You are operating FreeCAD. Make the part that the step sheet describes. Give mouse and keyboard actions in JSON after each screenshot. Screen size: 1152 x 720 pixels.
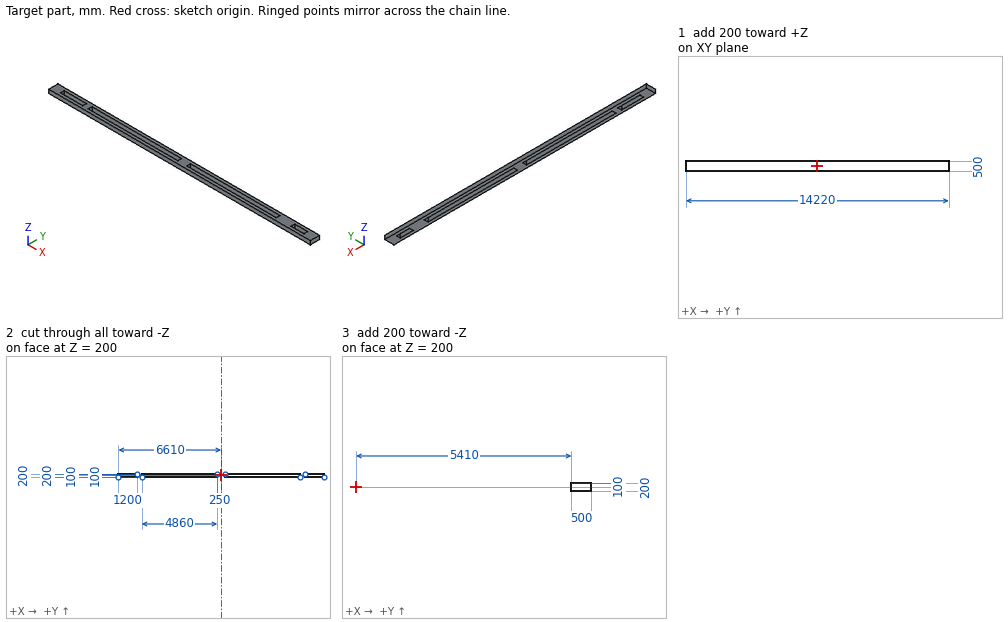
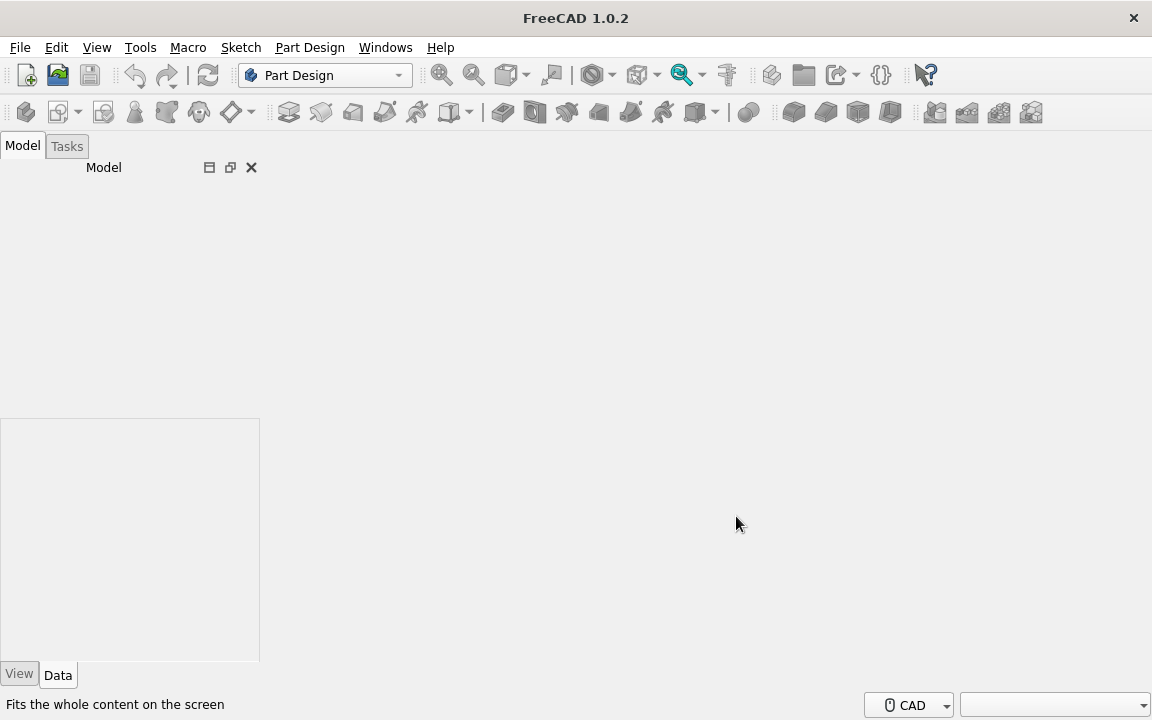
{"action": "left_click", "coordinate": [26, 76]}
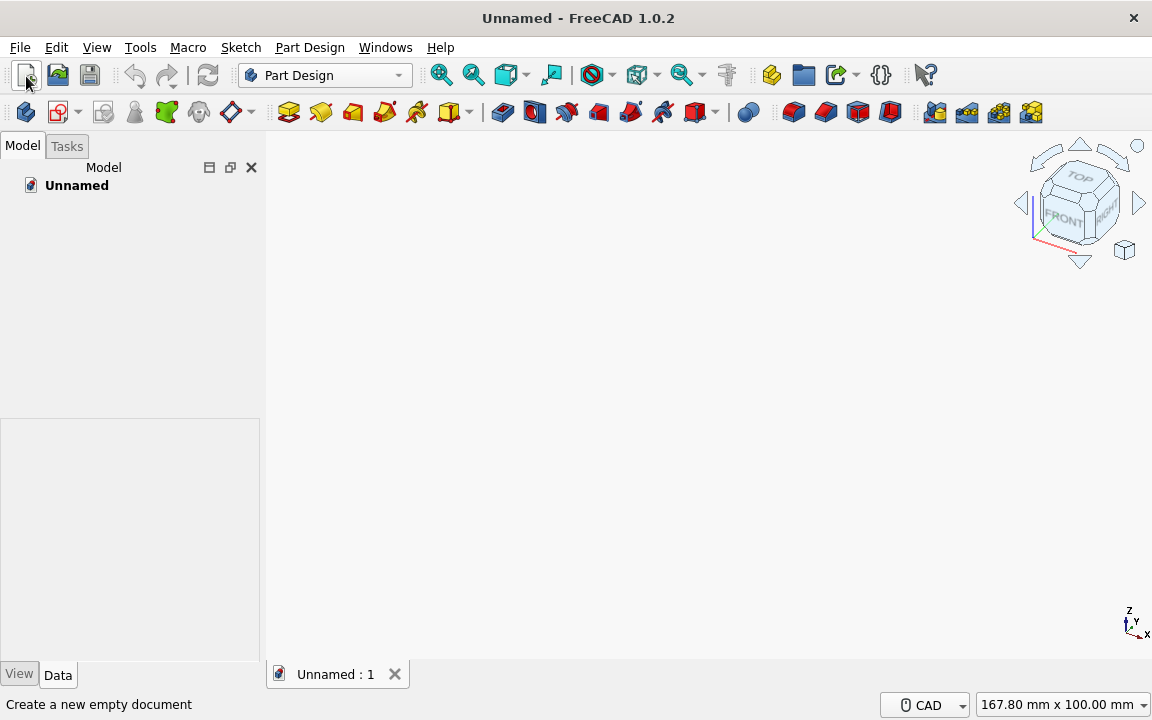
{"action": "left_click", "coordinate": [58, 112]}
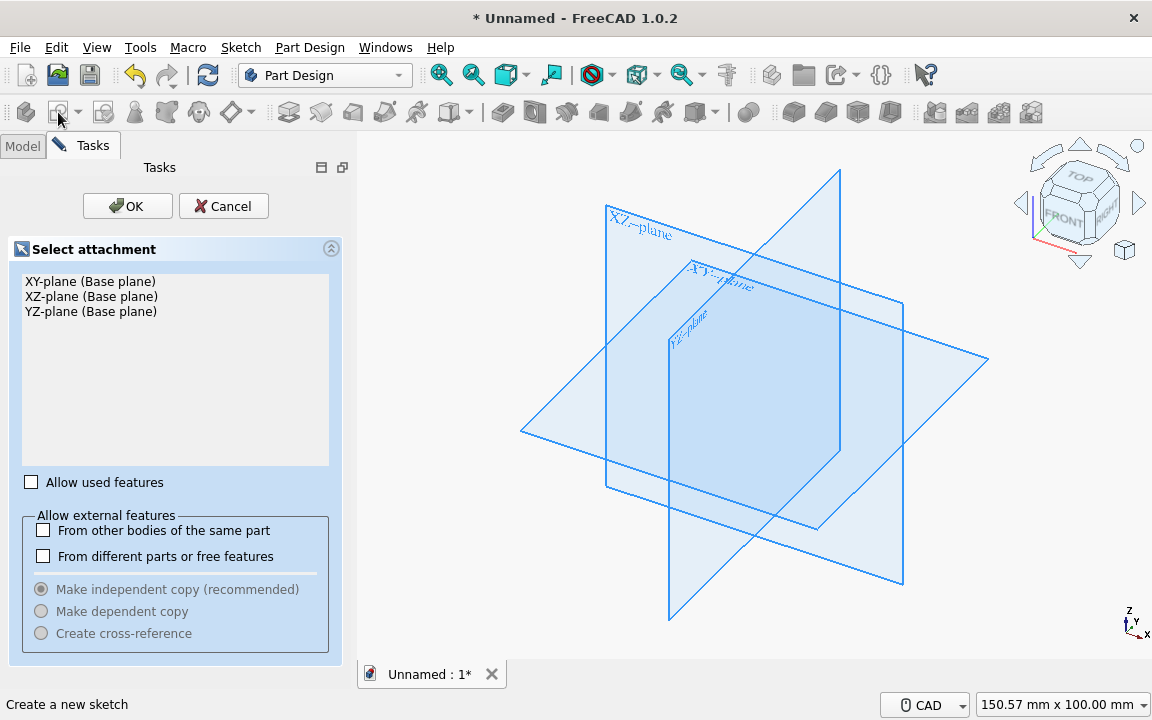
{"action": "left_click", "coordinate": [82, 282]}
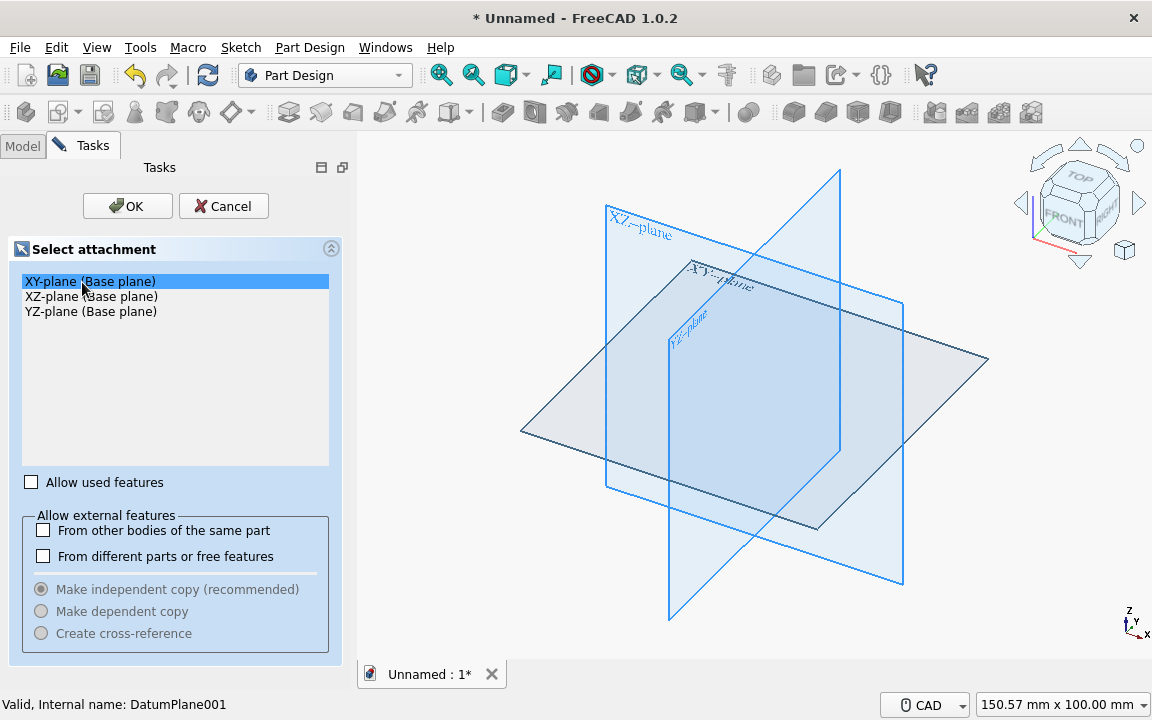
{"action": "left_click", "coordinate": [128, 206]}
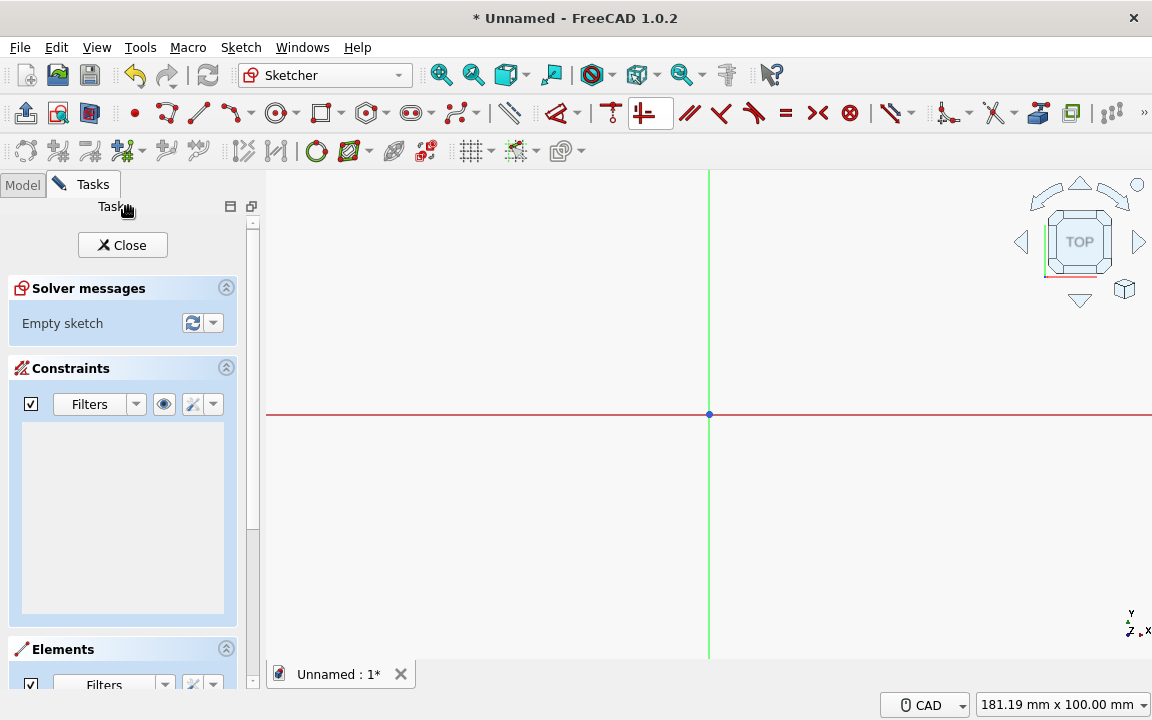
{"action": "scroll", "coordinate": [640, 414], "scroll_direction": "down", "scroll_amount": 15}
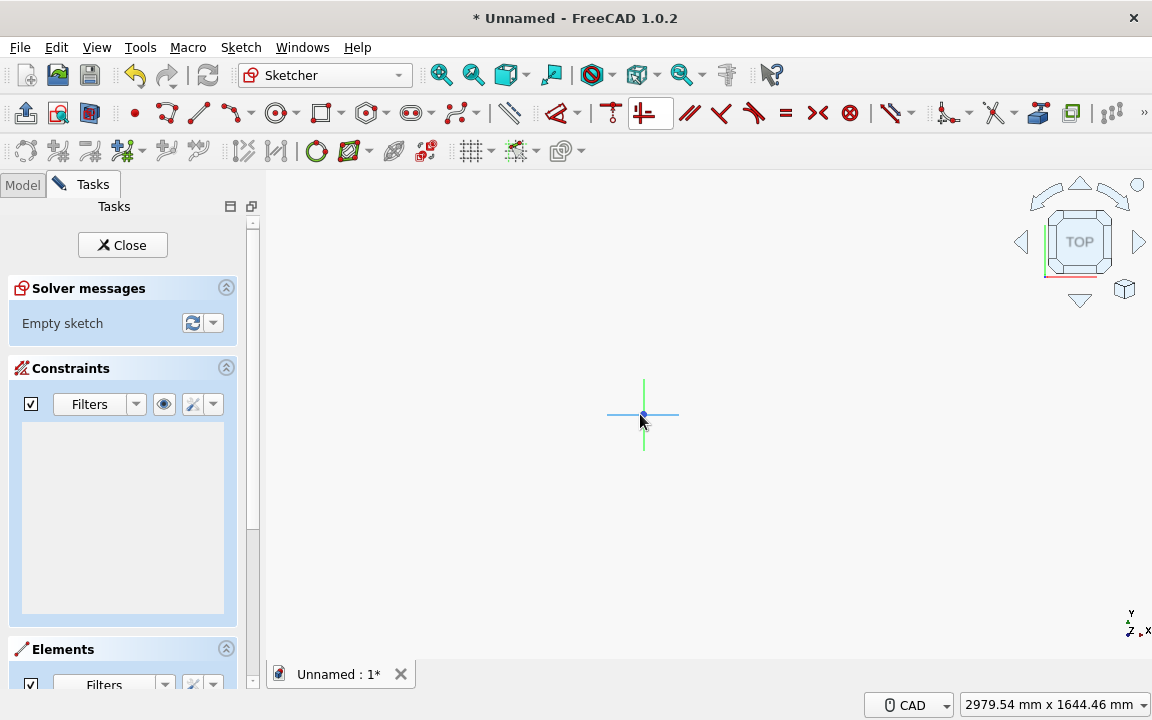
{"action": "scroll", "coordinate": [640, 414], "scroll_direction": "down", "scroll_amount": 10}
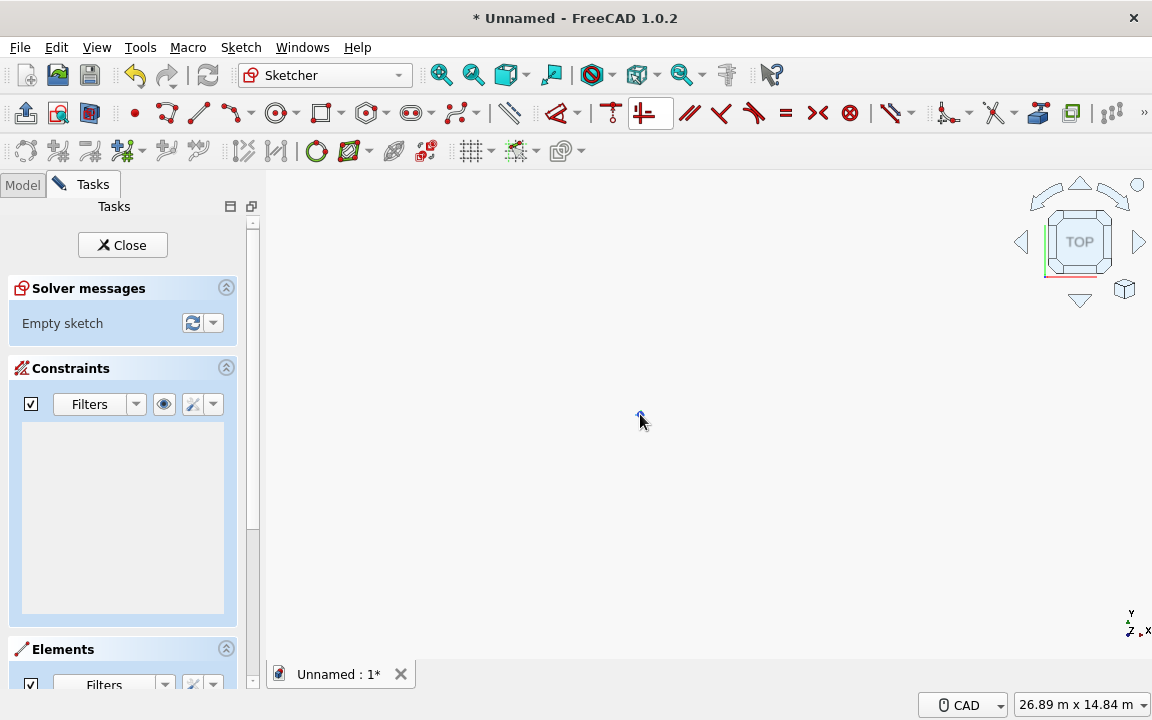
{"action": "left_click", "coordinate": [344, 114]}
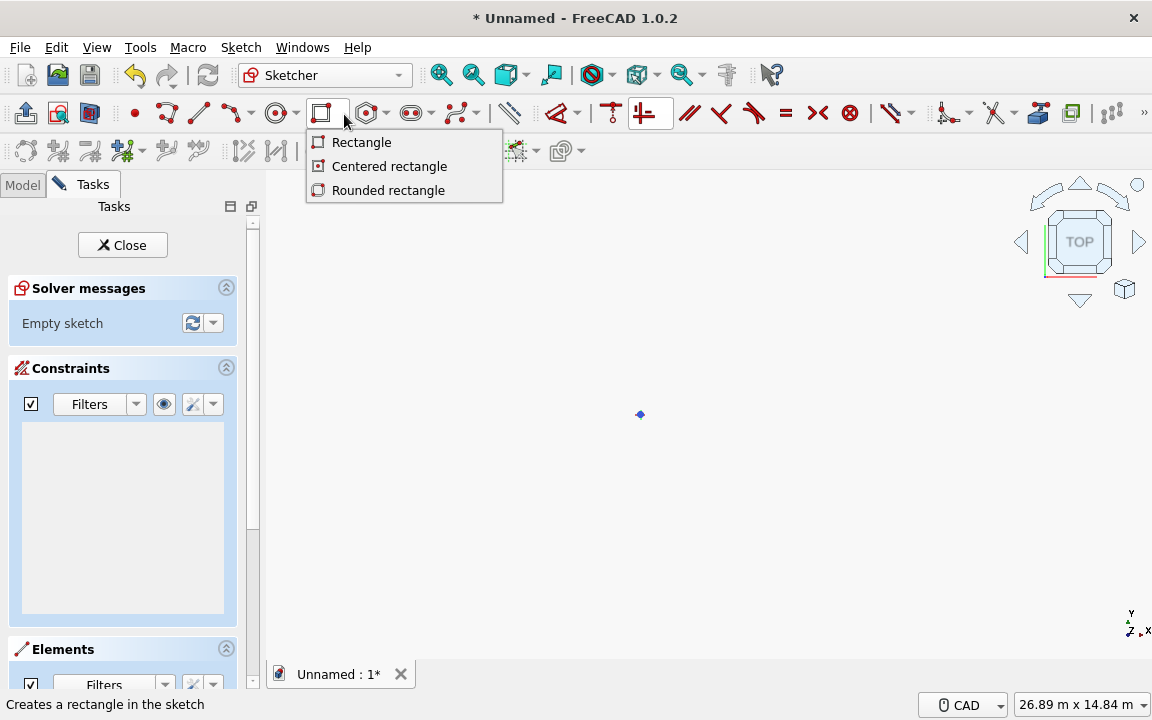
{"action": "left_click", "coordinate": [404, 166]}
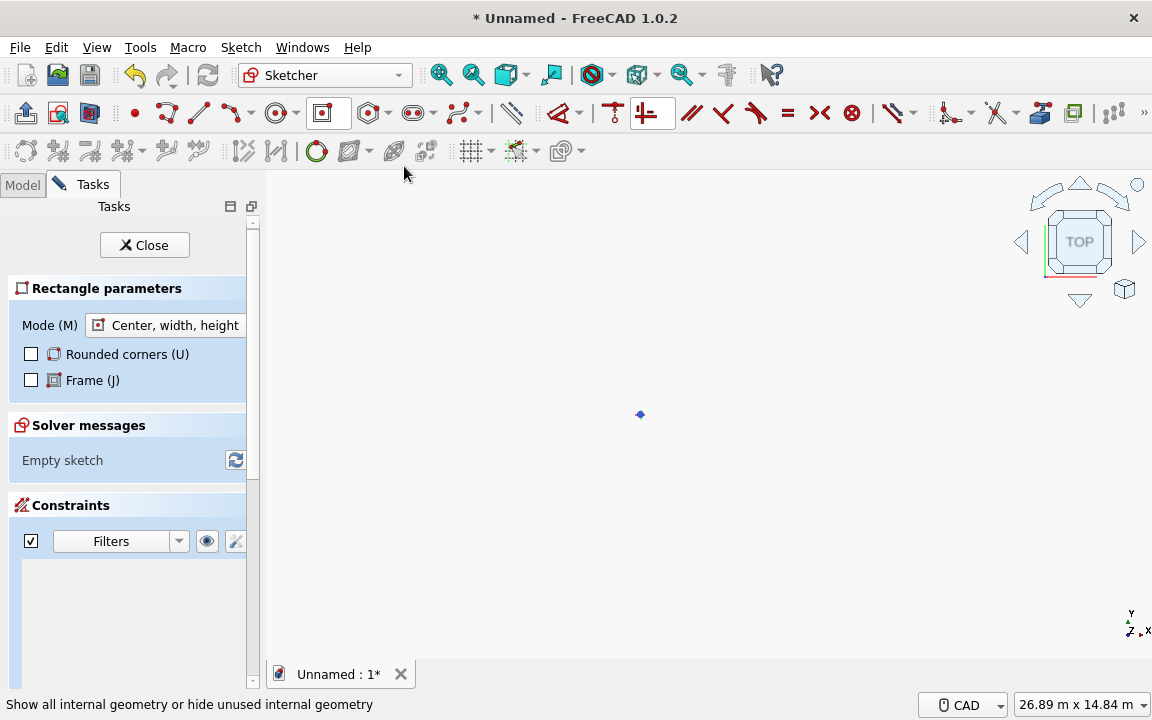
{"action": "scroll", "coordinate": [641, 414], "scroll_direction": "up", "scroll_amount": 4}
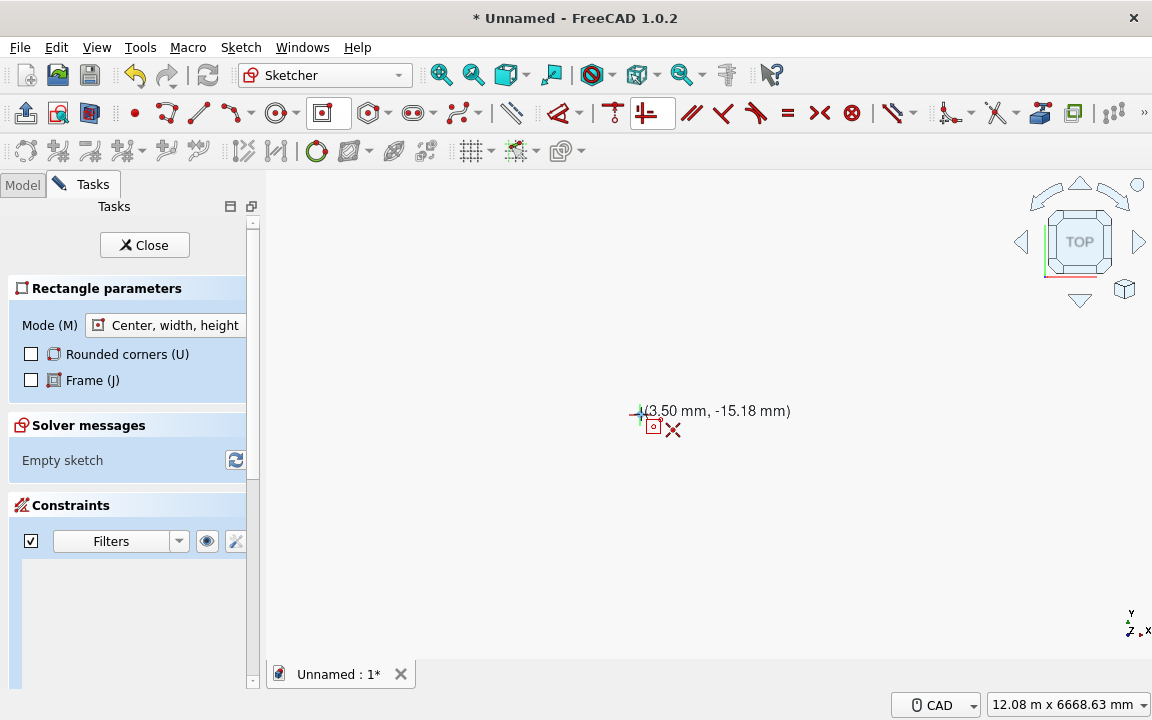
{"action": "left_click", "coordinate": [640, 414]}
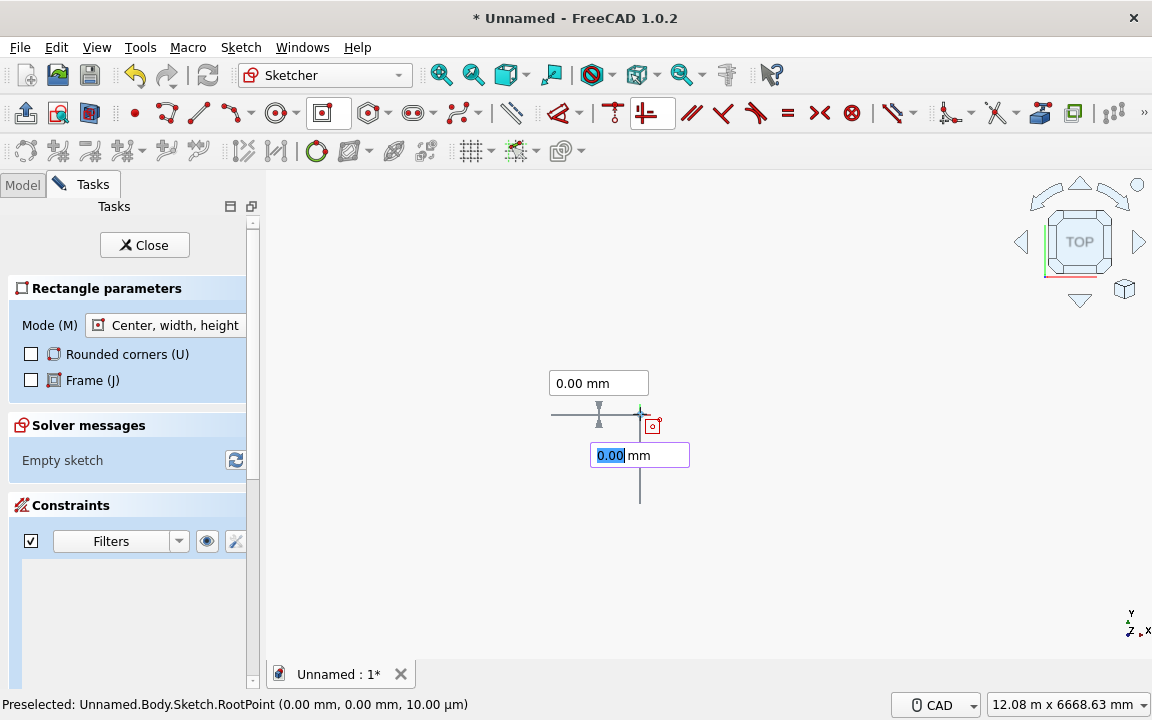
{"action": "scroll", "coordinate": [641, 414], "scroll_direction": "down", "scroll_amount": 4}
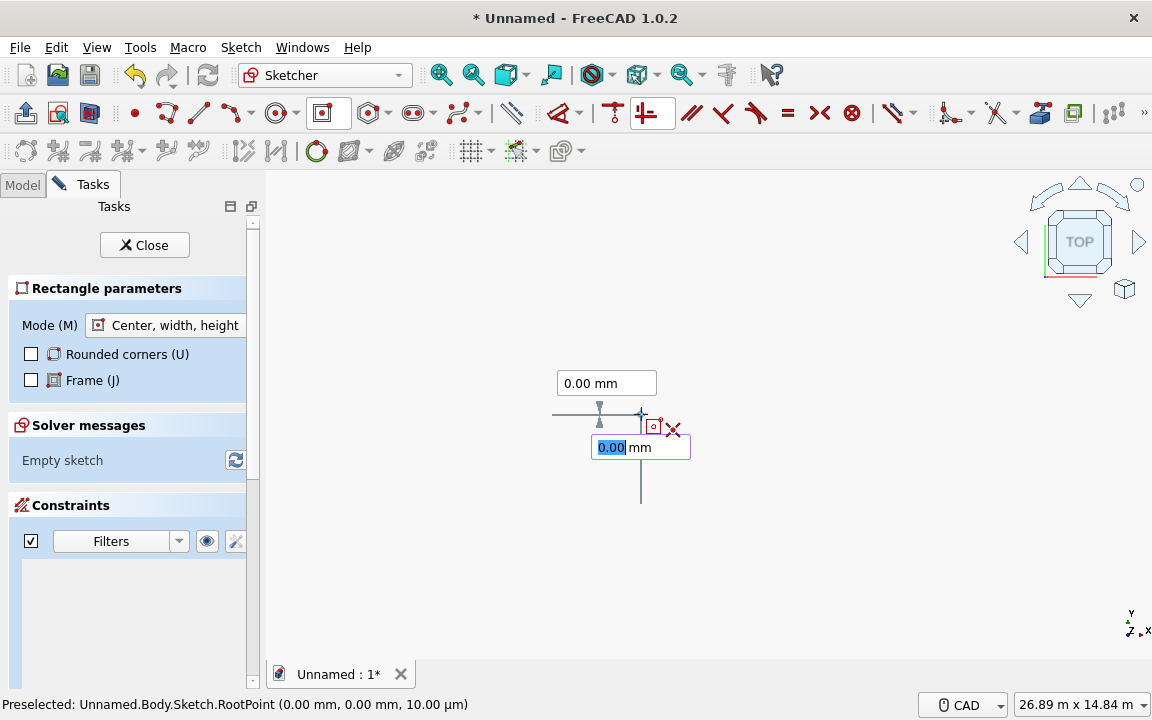
{"action": "scroll", "coordinate": [875, 406], "scroll_direction": "up", "scroll_amount": 4}